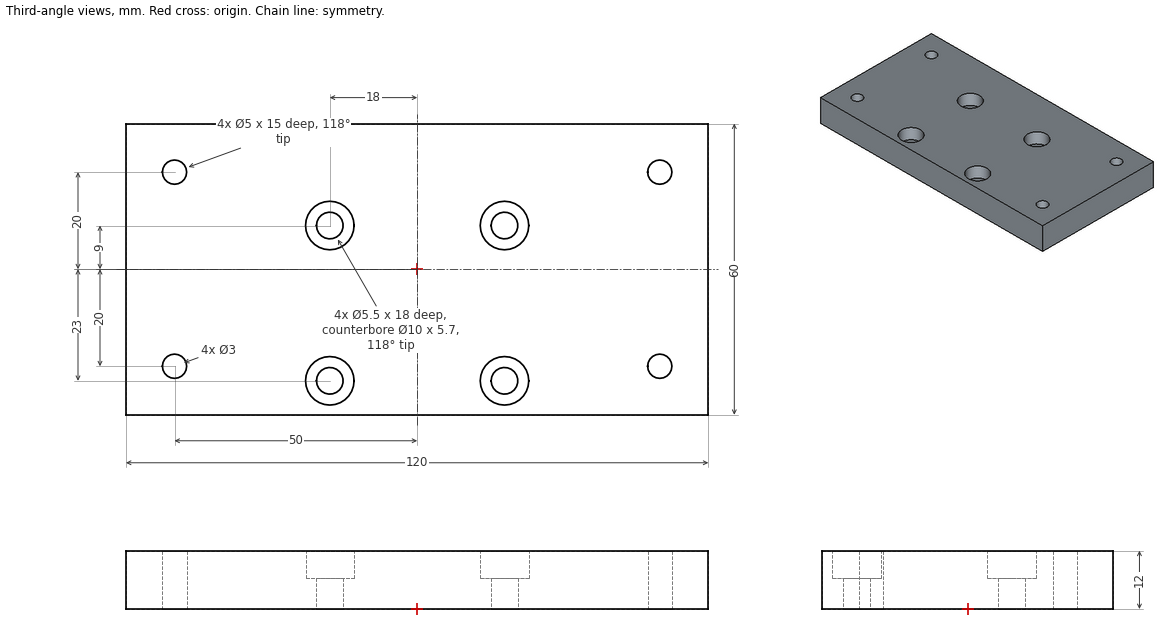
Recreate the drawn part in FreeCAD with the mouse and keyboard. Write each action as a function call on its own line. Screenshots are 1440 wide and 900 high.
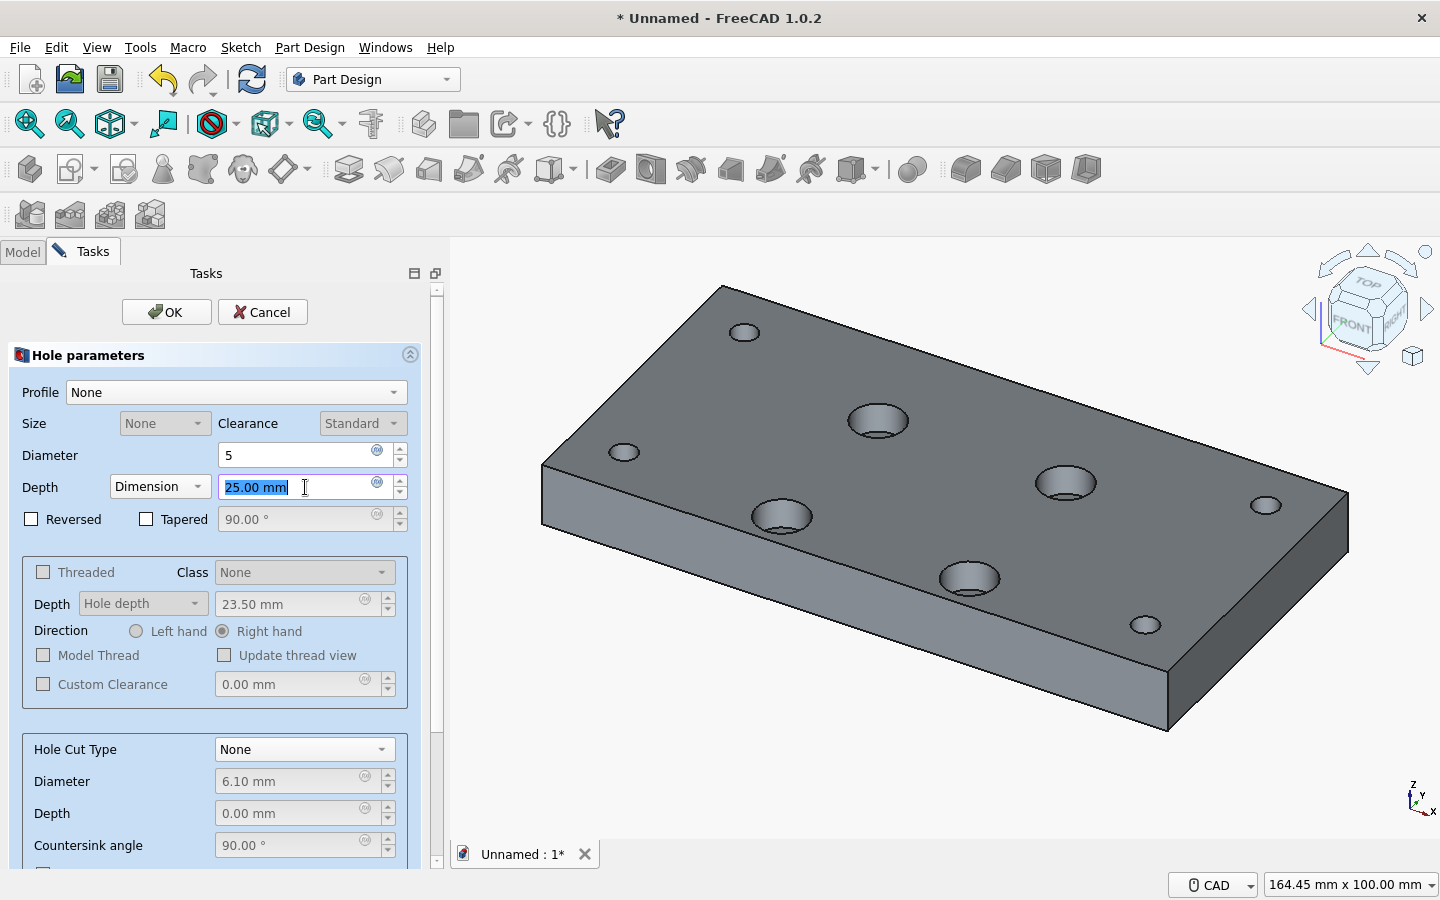
text(15)
key(Tab)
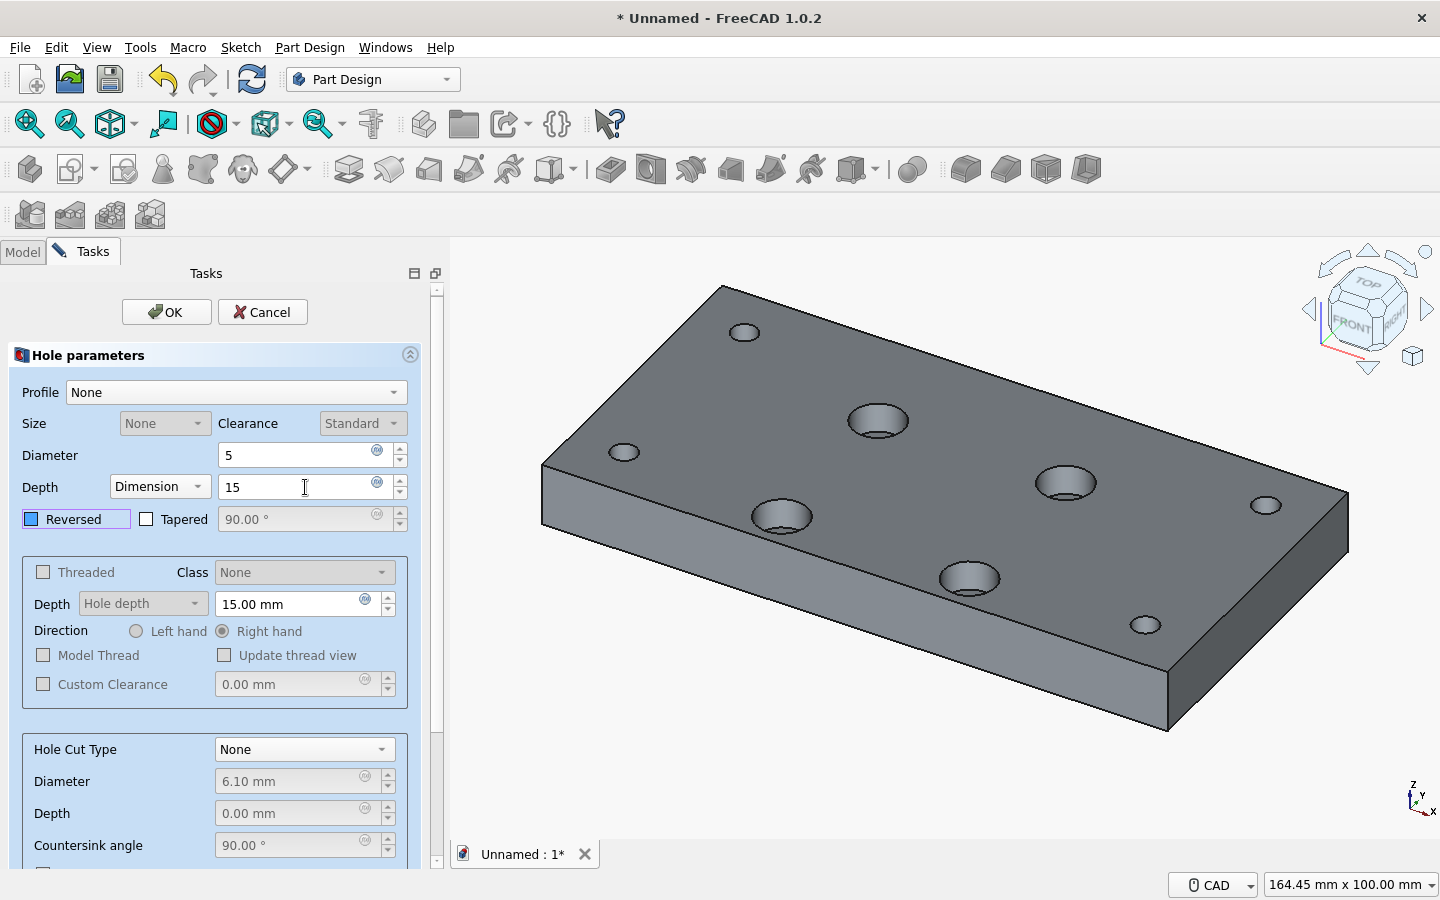
click(167, 312)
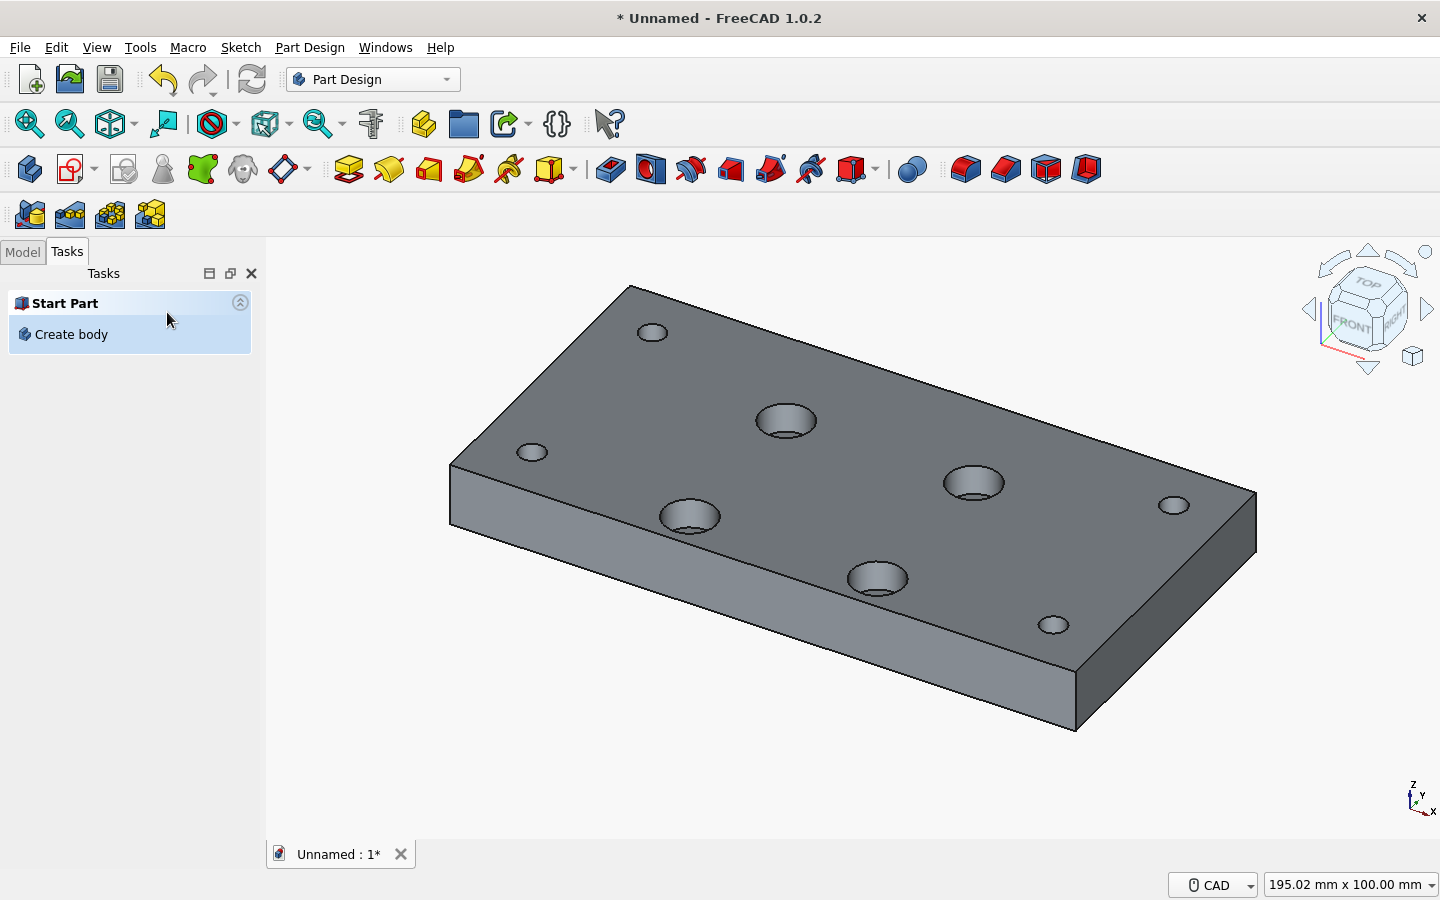
key(0)